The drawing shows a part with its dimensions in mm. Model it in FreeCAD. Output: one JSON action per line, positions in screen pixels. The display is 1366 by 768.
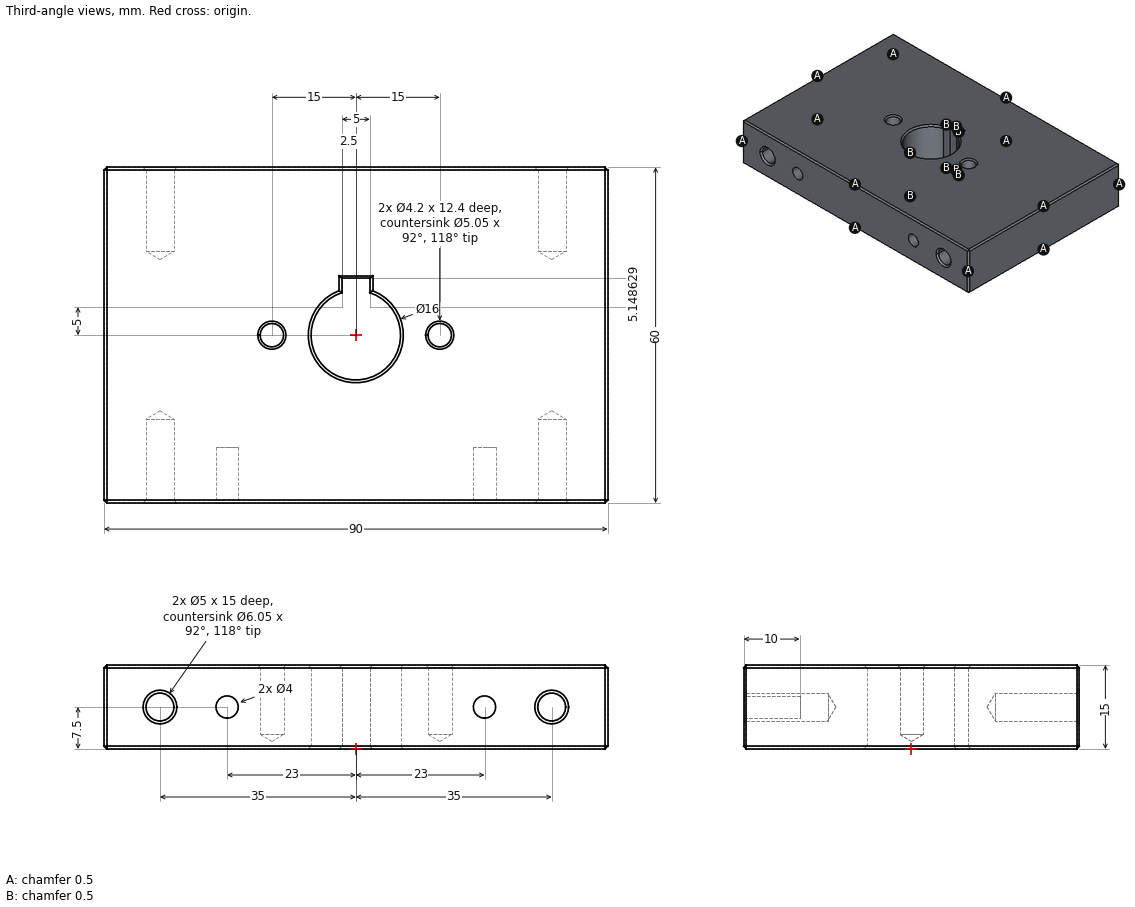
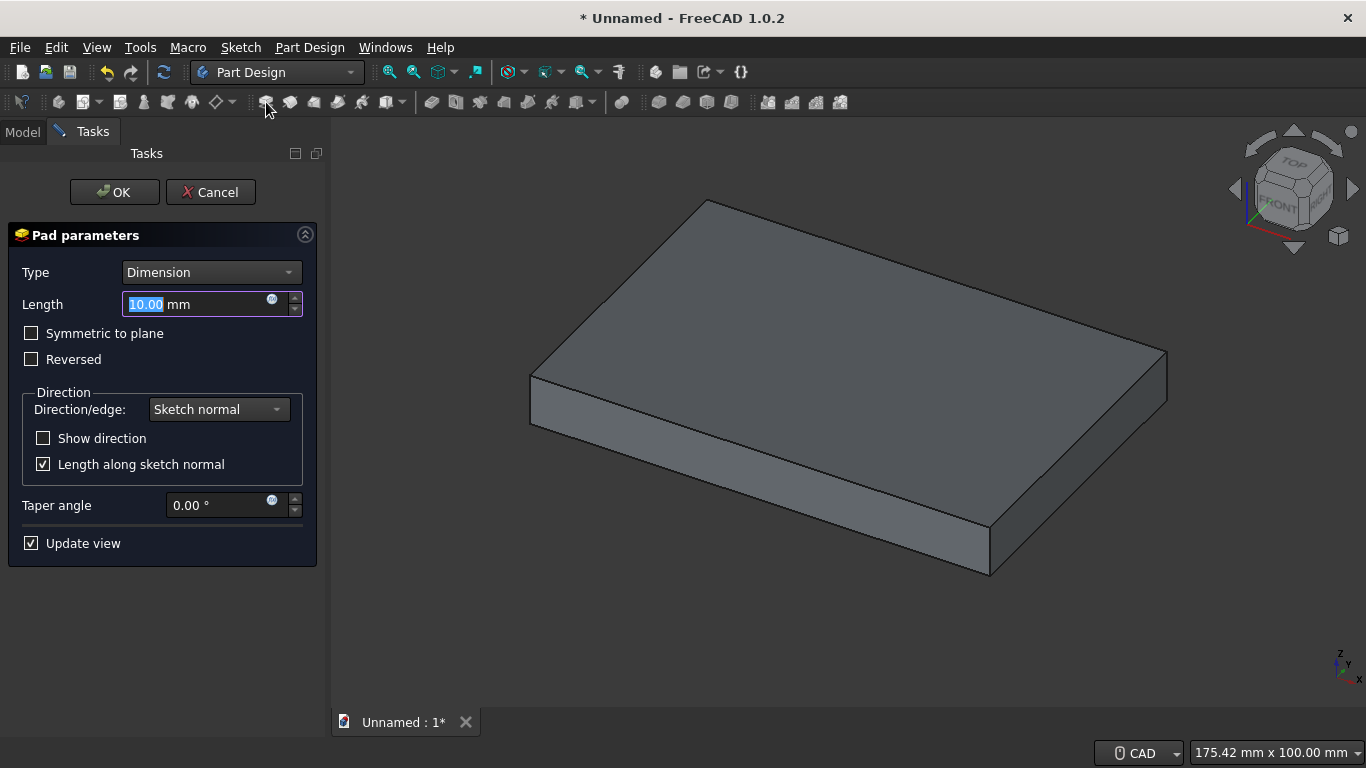
{"action": "type", "text": "15"}
{"action": "key", "text": "Tab"}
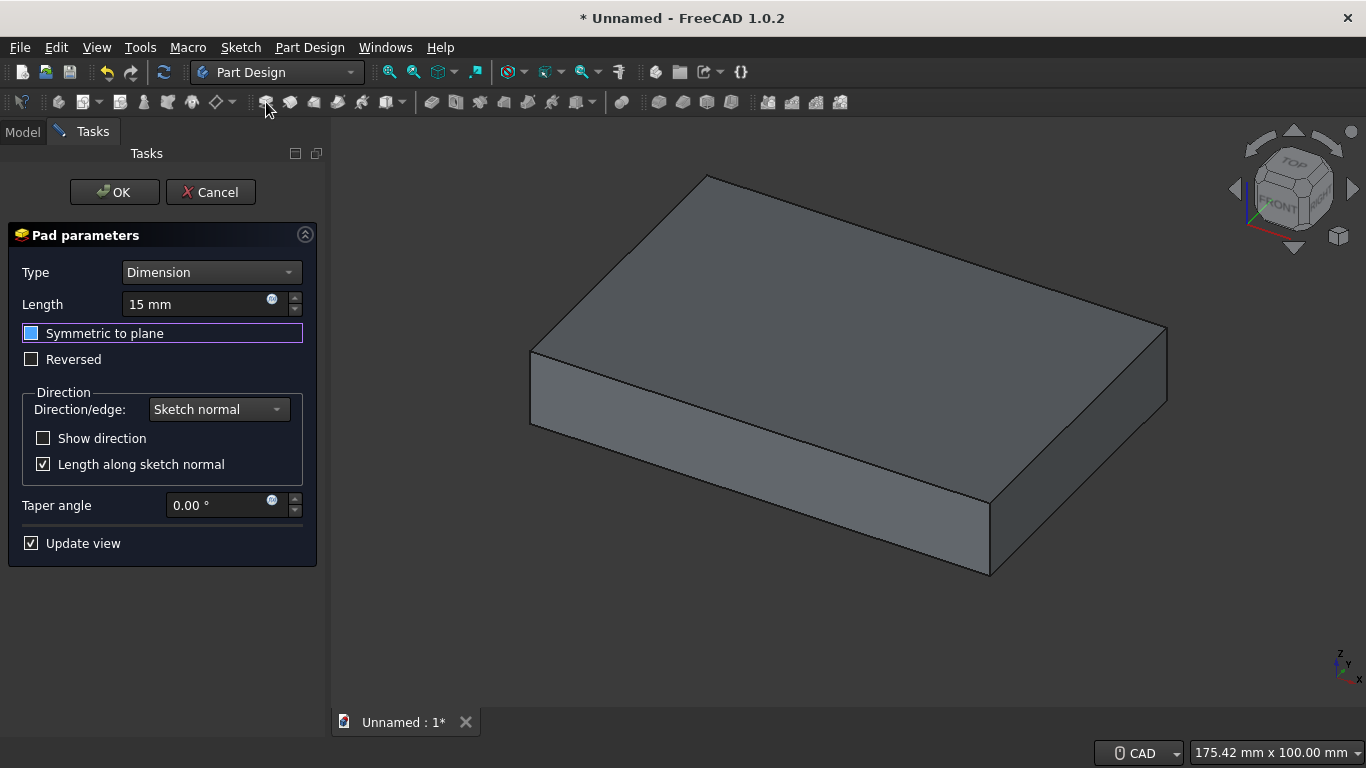
{"action": "left_click", "coordinate": [115, 192]}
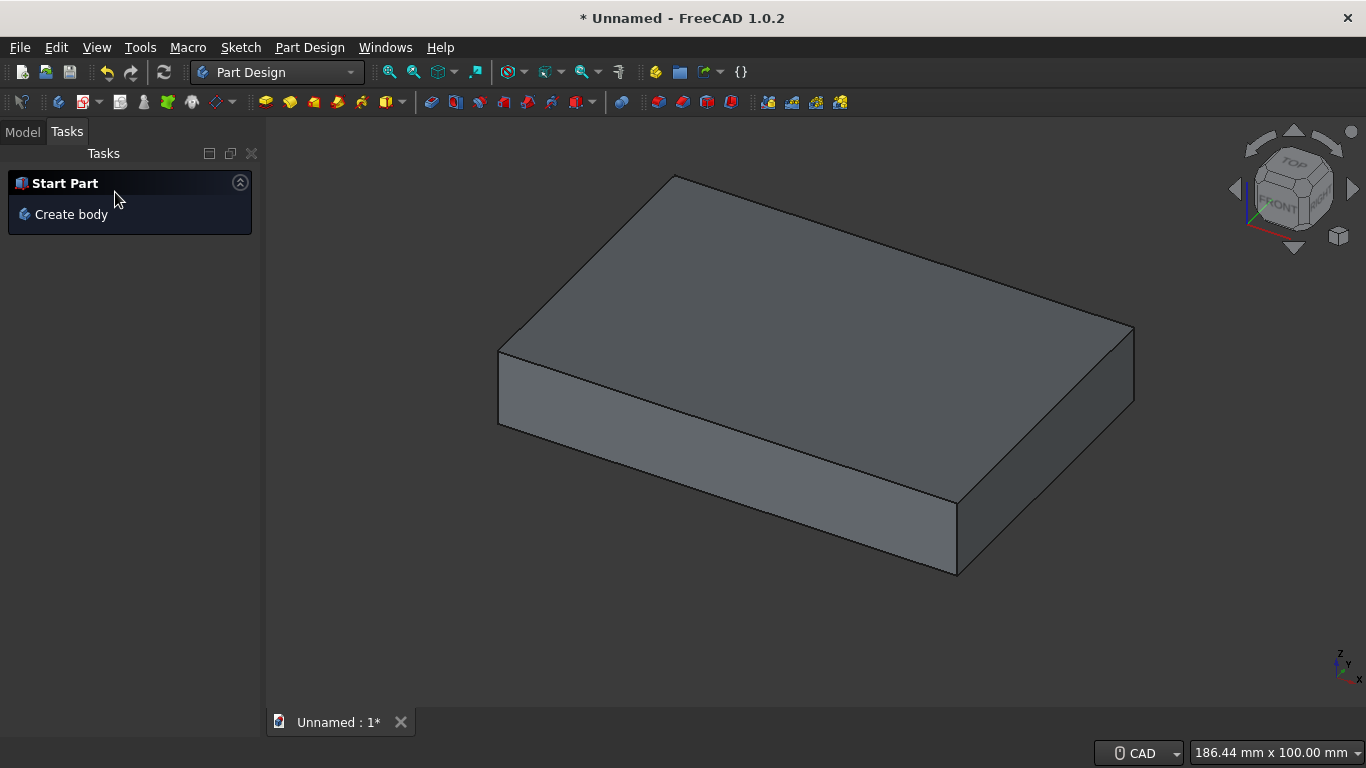
{"action": "left_click", "coordinate": [882, 360]}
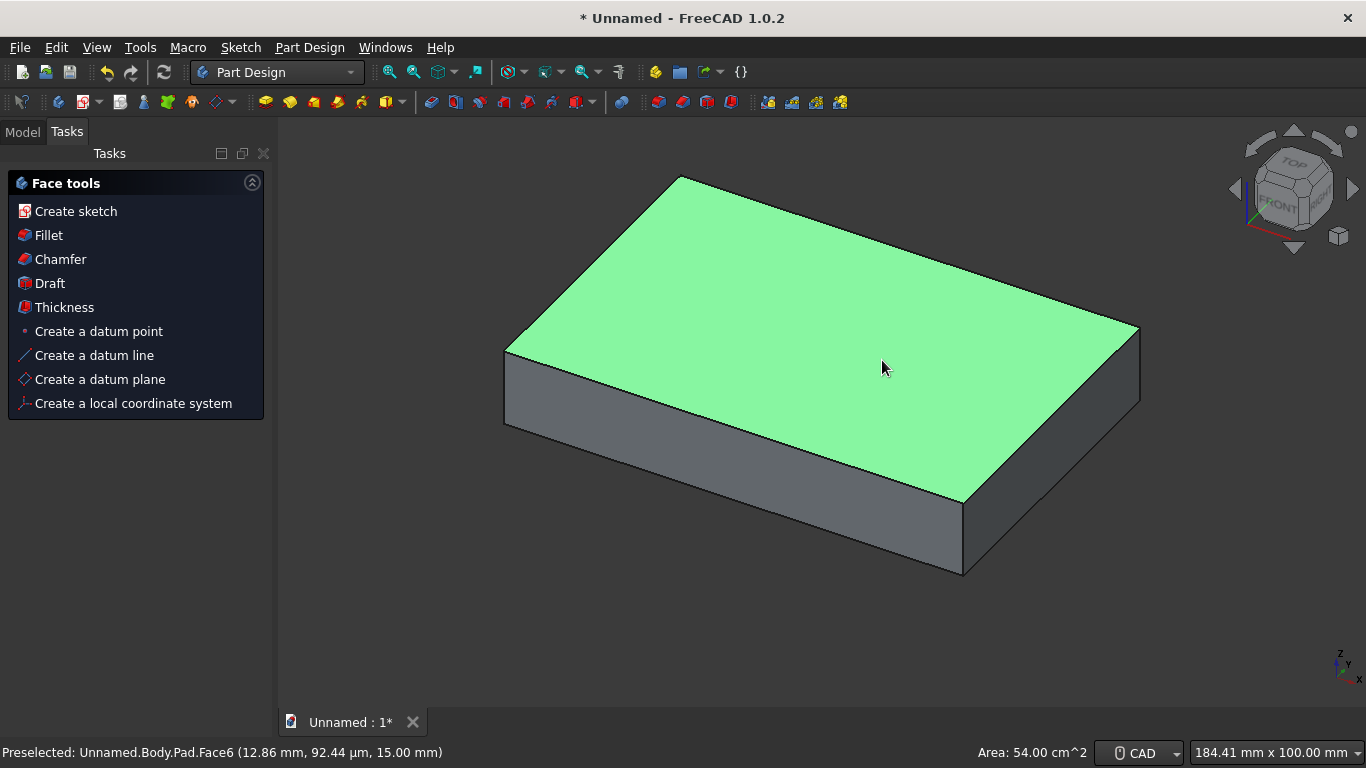
{"action": "left_click", "coordinate": [84, 102]}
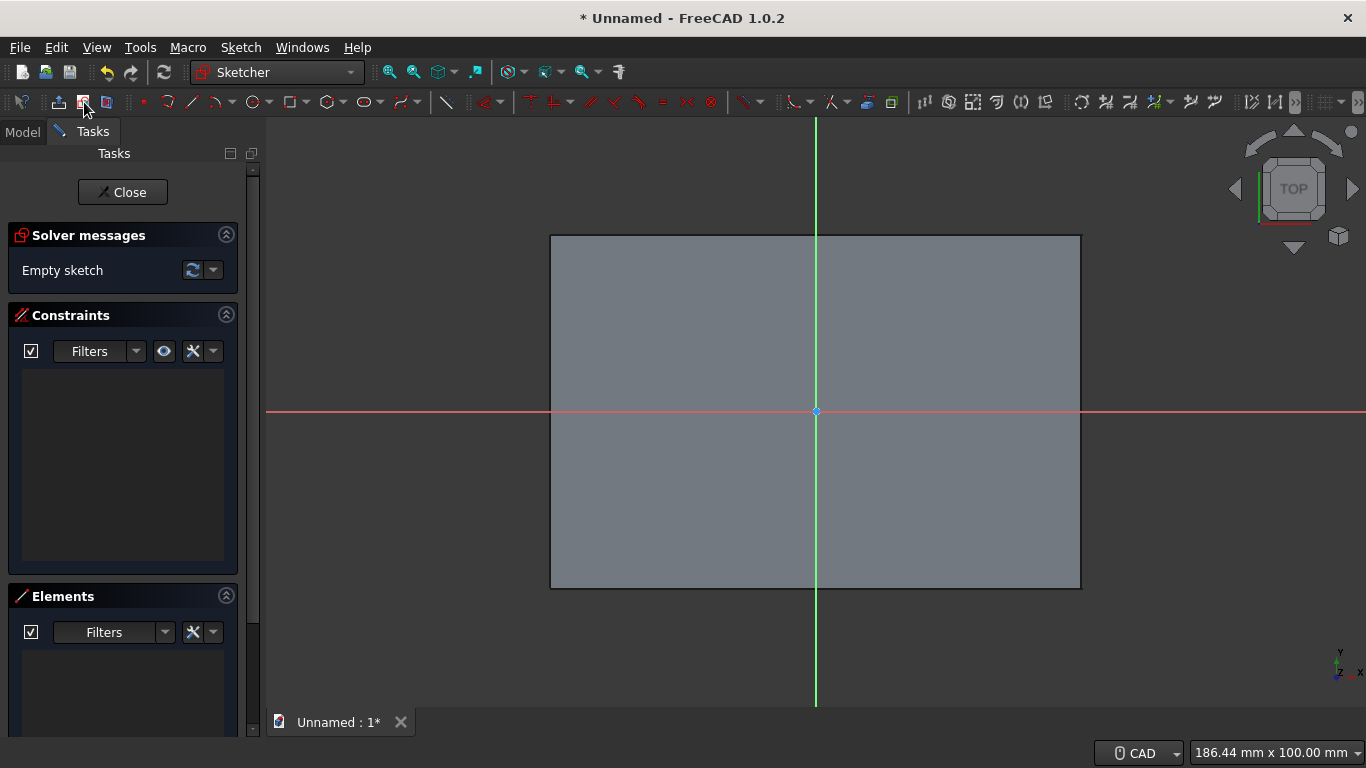
{"action": "scroll", "coordinate": [838, 412], "scroll_direction": "up", "scroll_amount": 7}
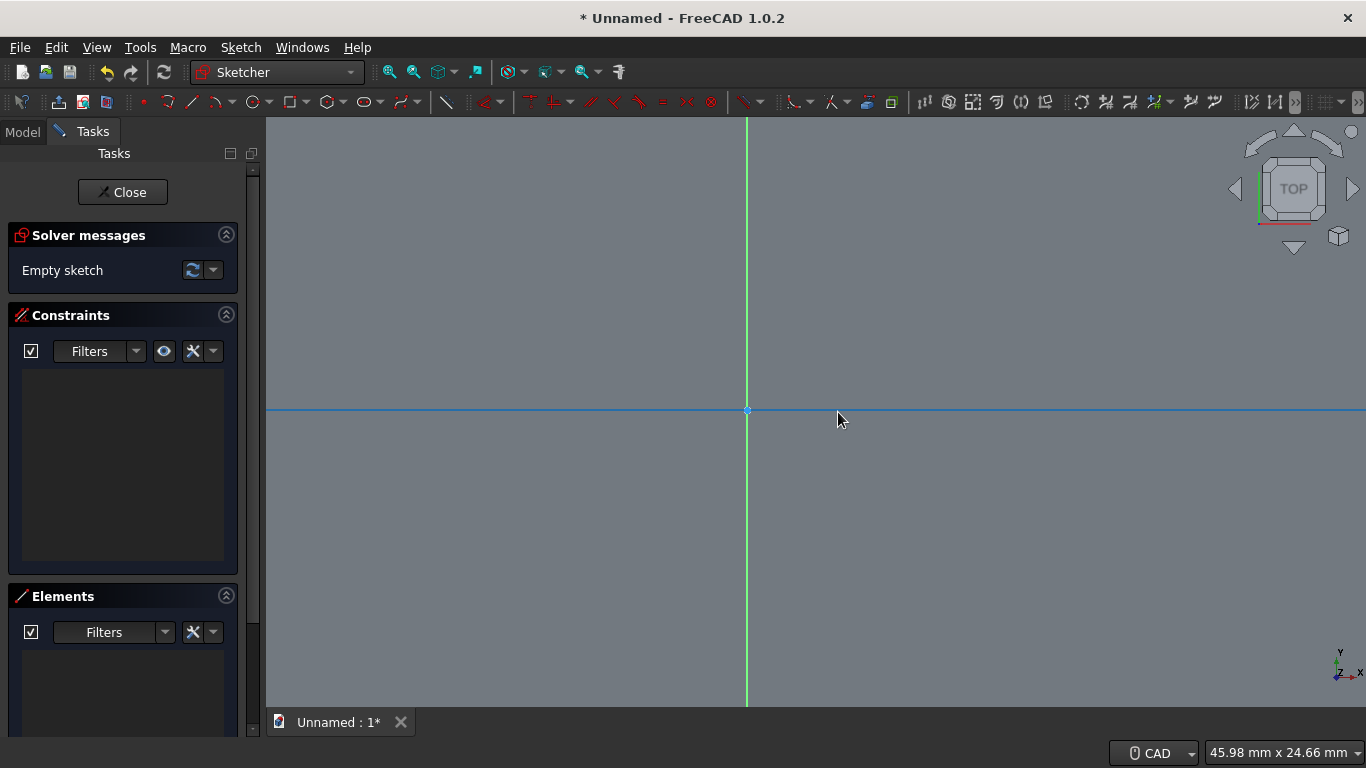
{"action": "key", "text": "g c"}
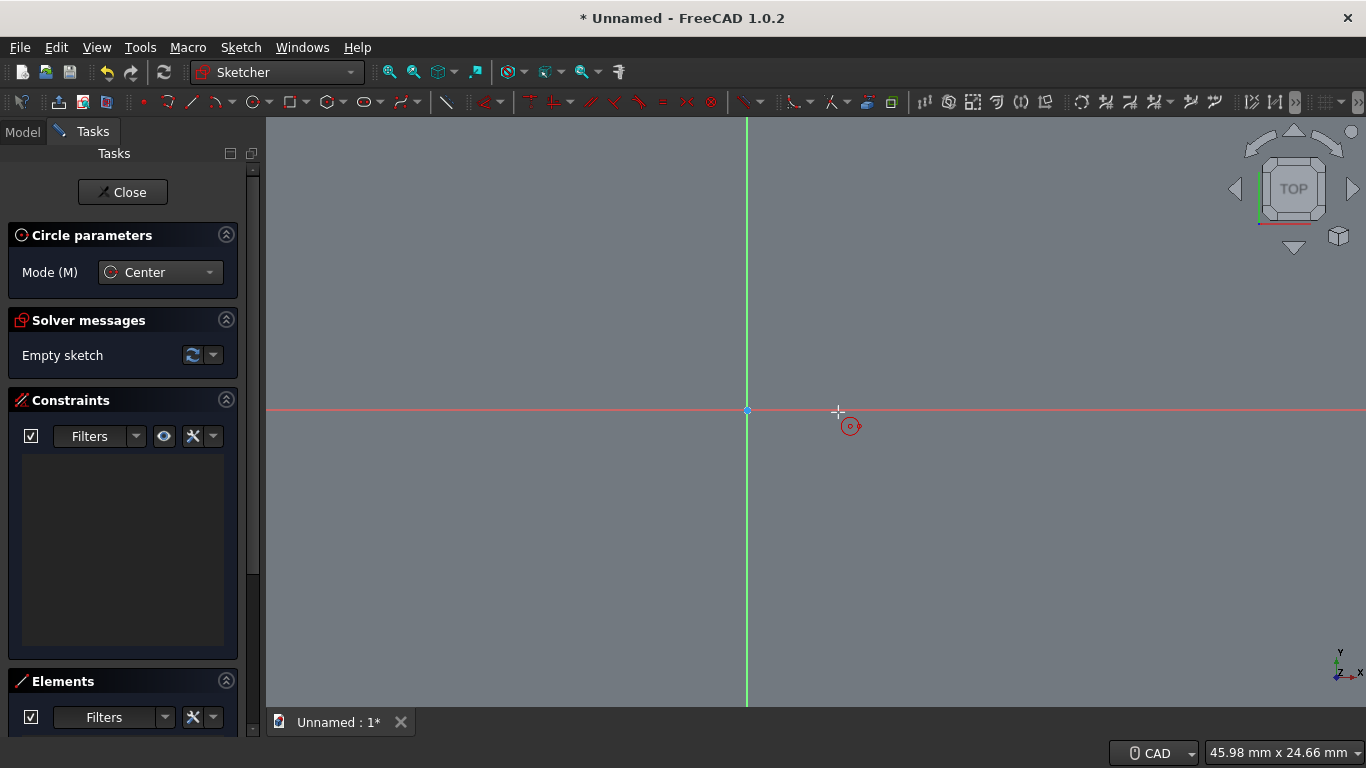
{"action": "left_click", "coordinate": [747, 410]}
{"action": "mouse_move", "coordinate": [883, 275]}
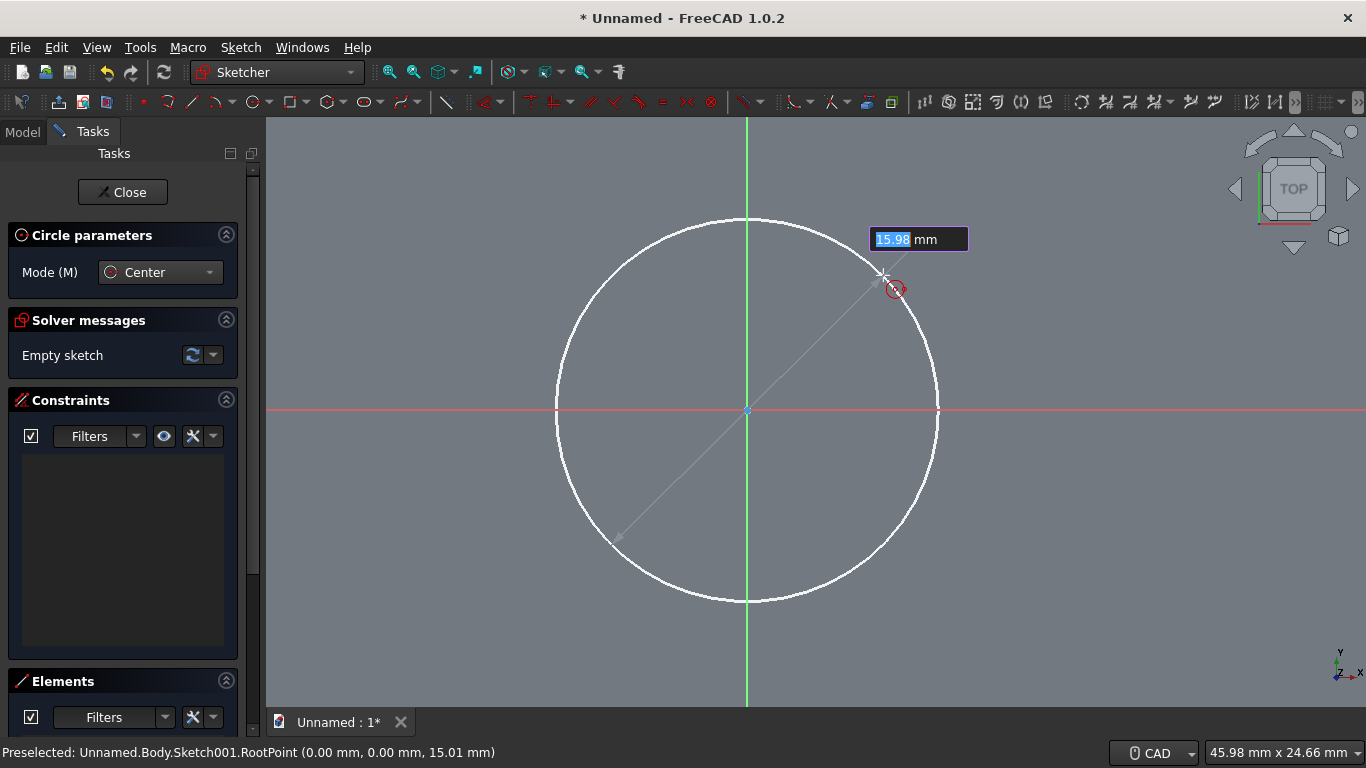
{"action": "type", "text": "16"}
{"action": "key", "text": "Return"}
{"action": "key", "text": "Escape"}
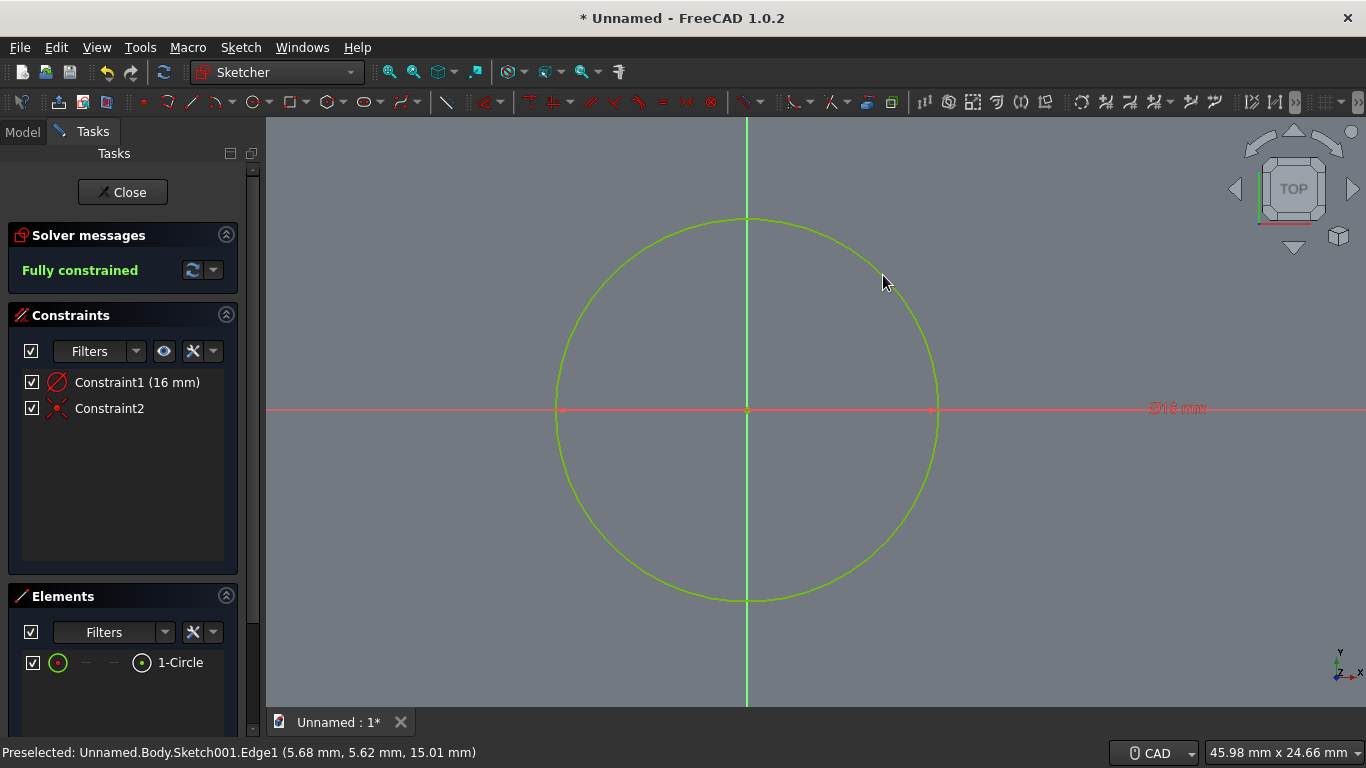
{"action": "left_click", "coordinate": [123, 192]}